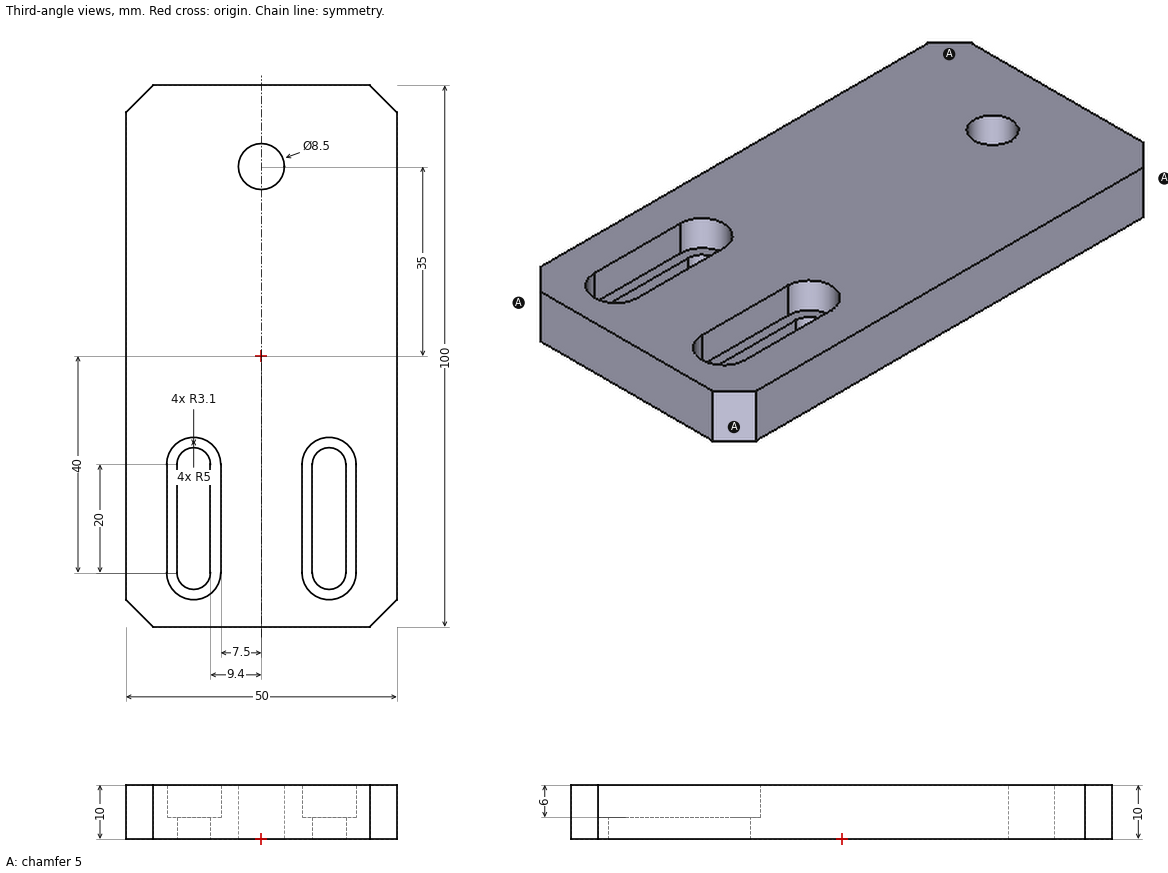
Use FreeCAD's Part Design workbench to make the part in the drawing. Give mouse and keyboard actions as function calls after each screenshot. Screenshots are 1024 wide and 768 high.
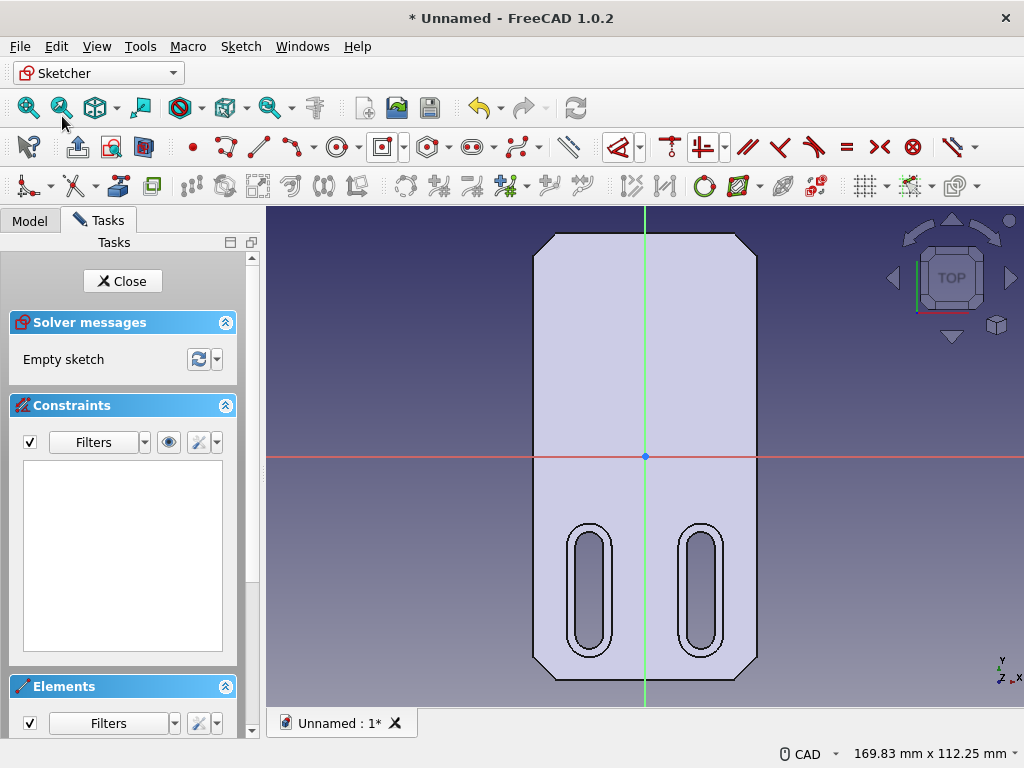
scroll(654, 281, up, 11)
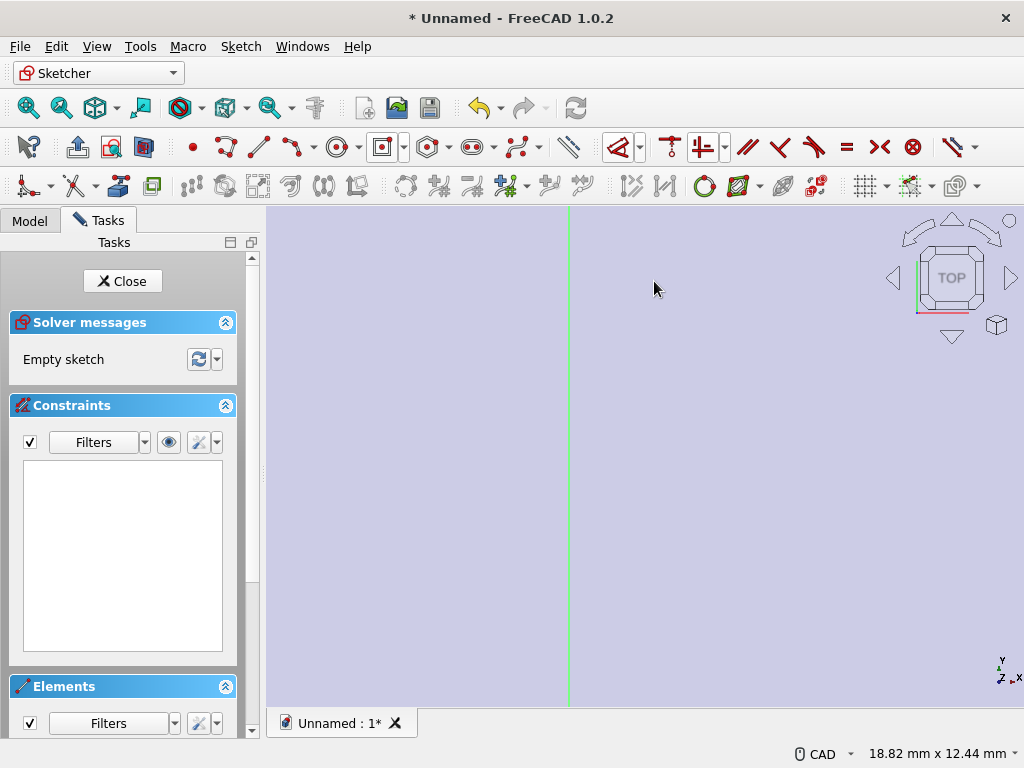
click(336, 148)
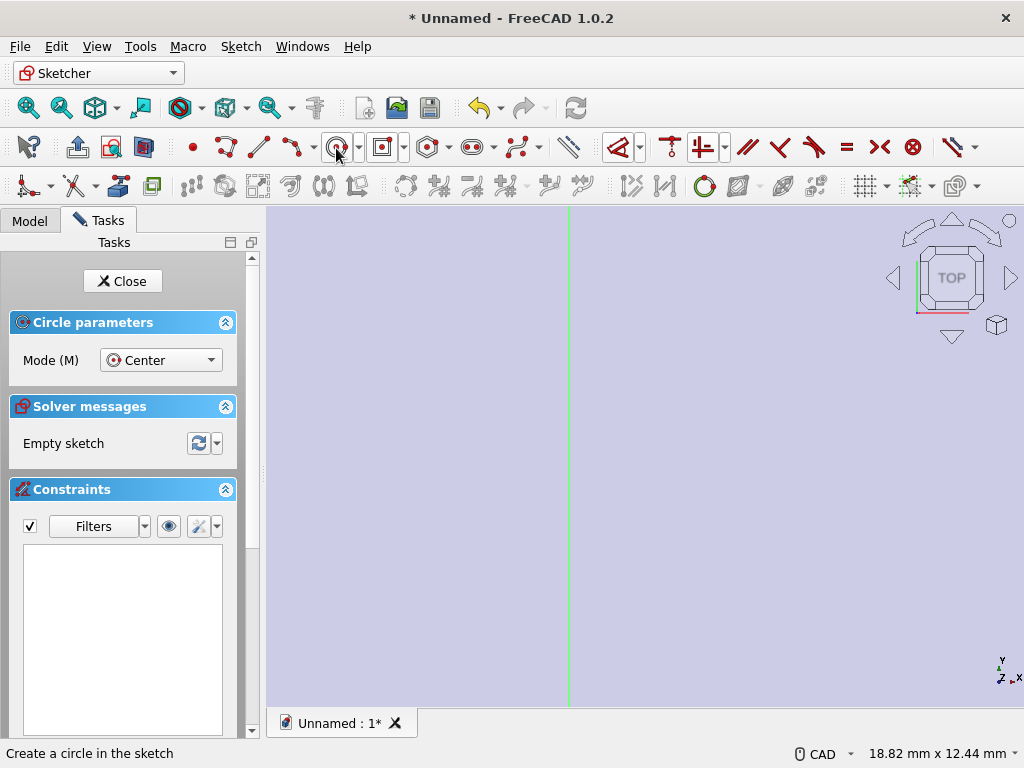
click(569, 454)
click(690, 333)
key(Escape)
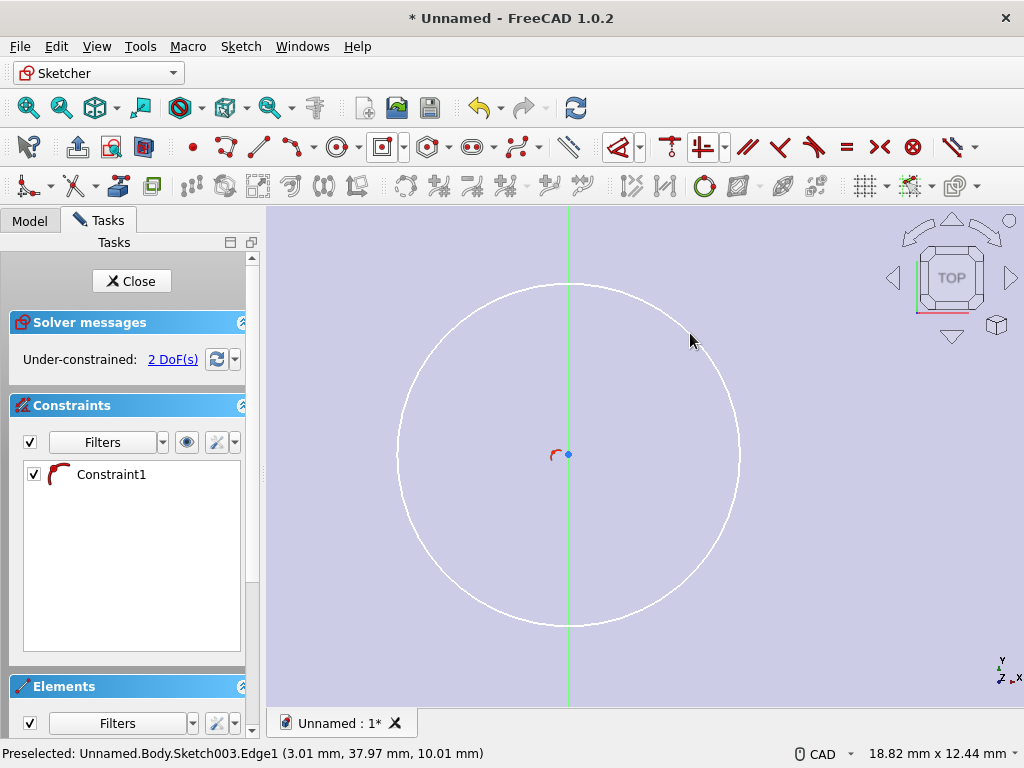
click(689, 333)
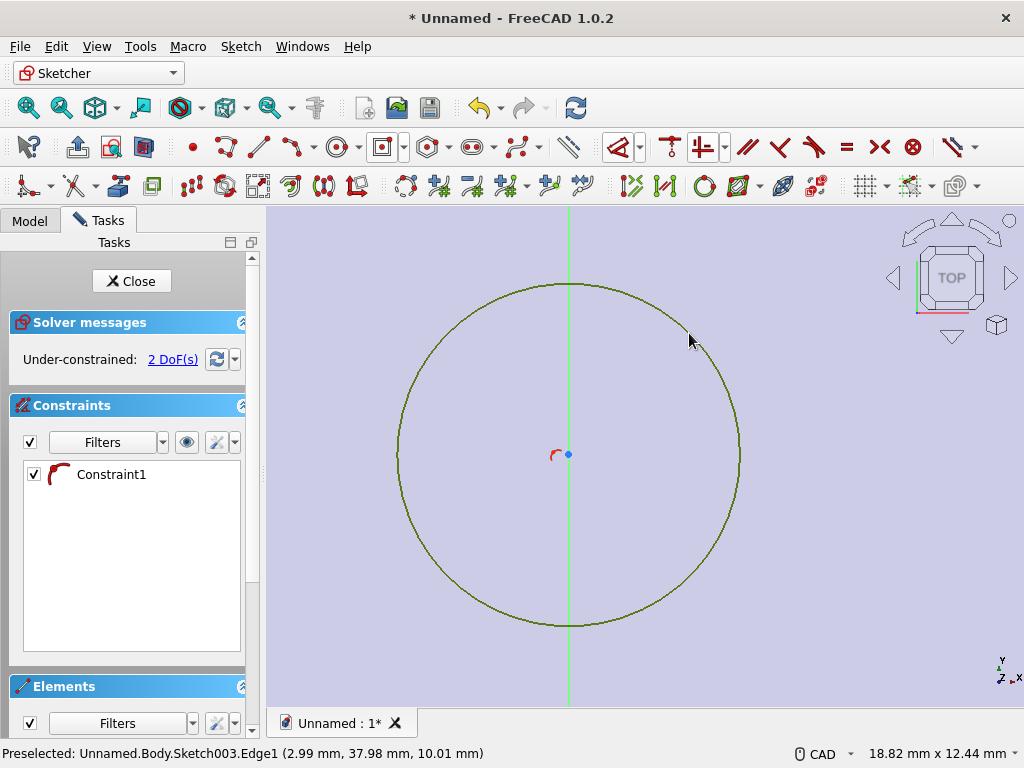
key(k)
key(o)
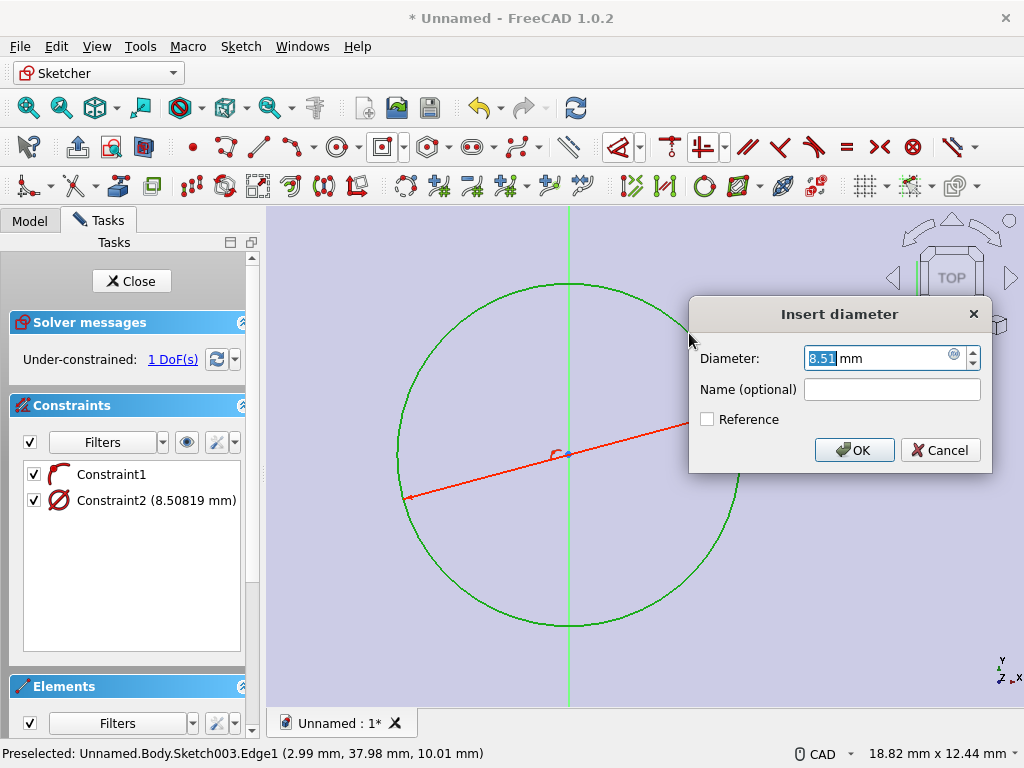
text(8.5)
key(Return)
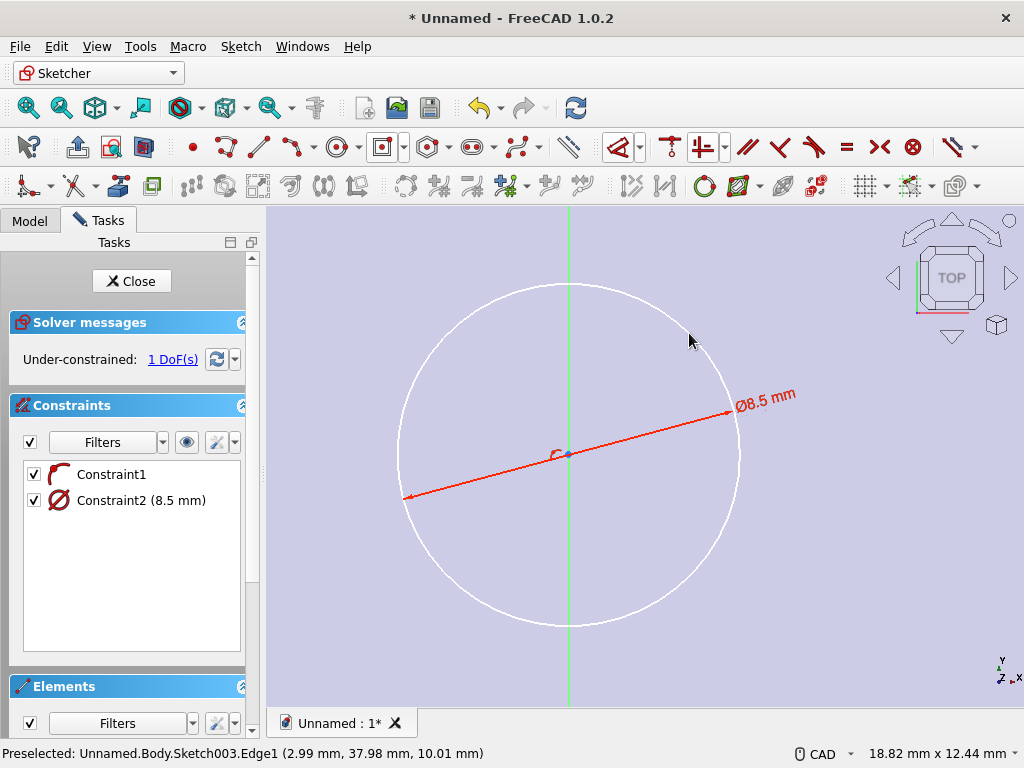
click(569, 455)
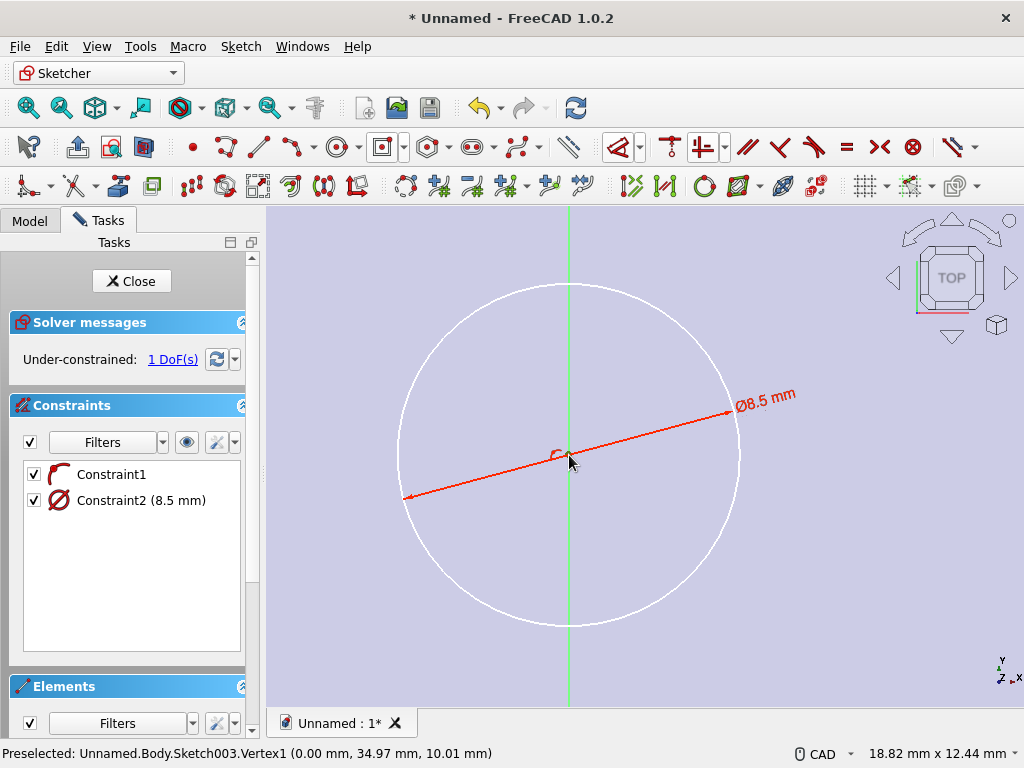
key(i)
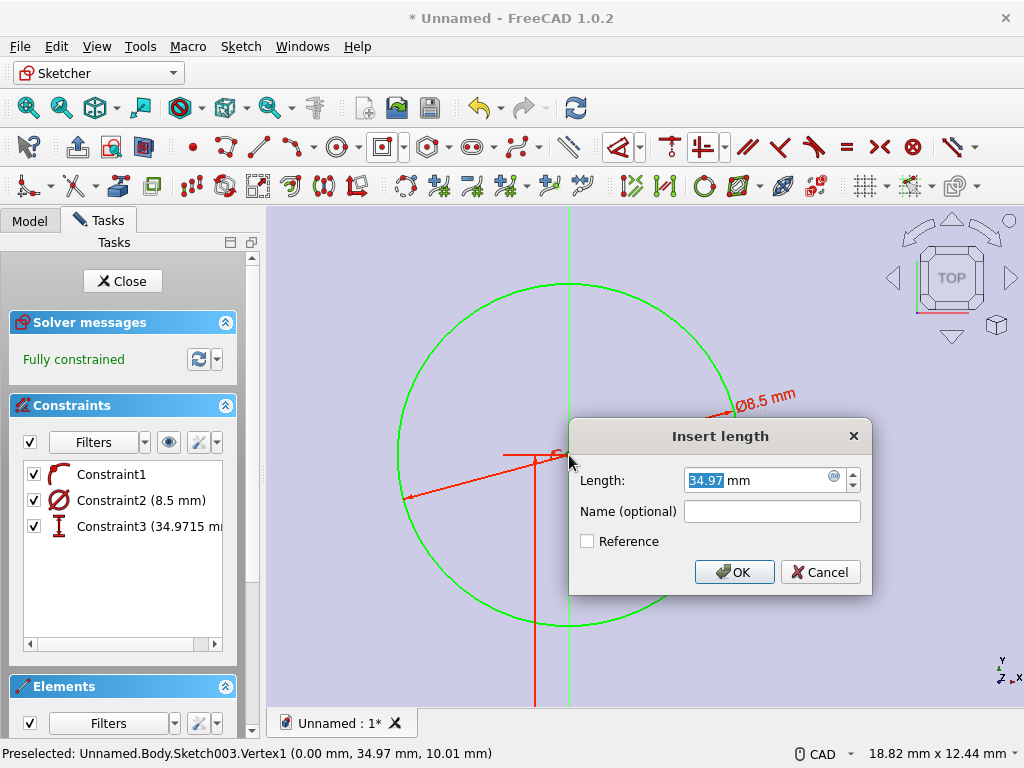
text(35)
key(Return)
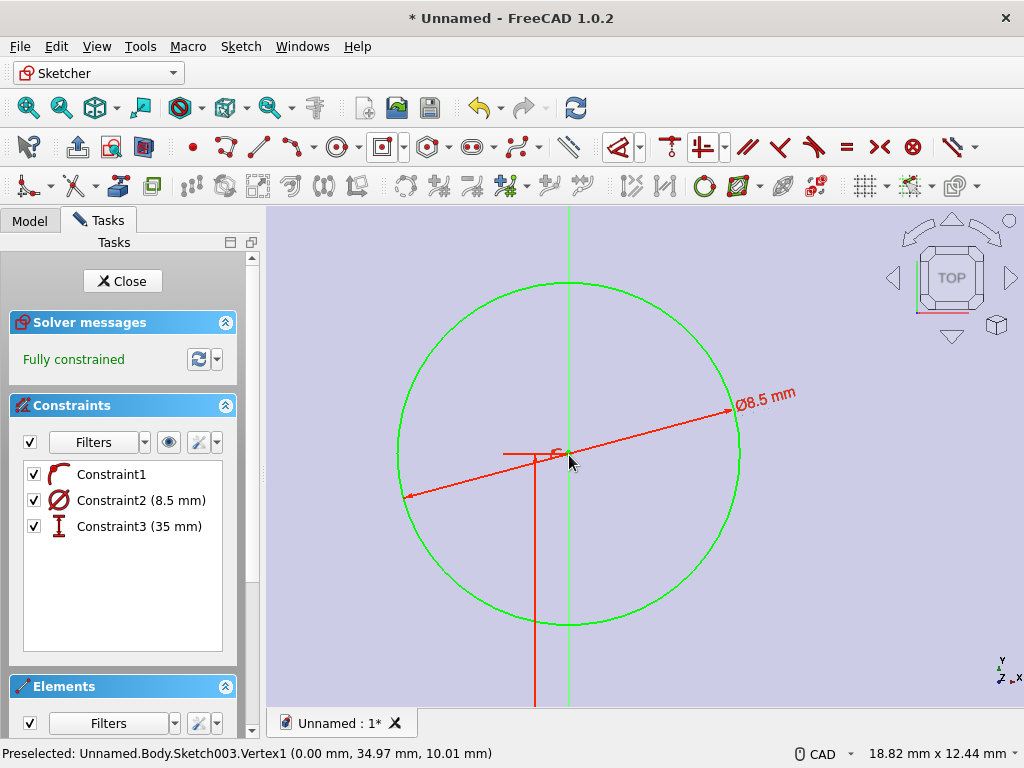
click(123, 281)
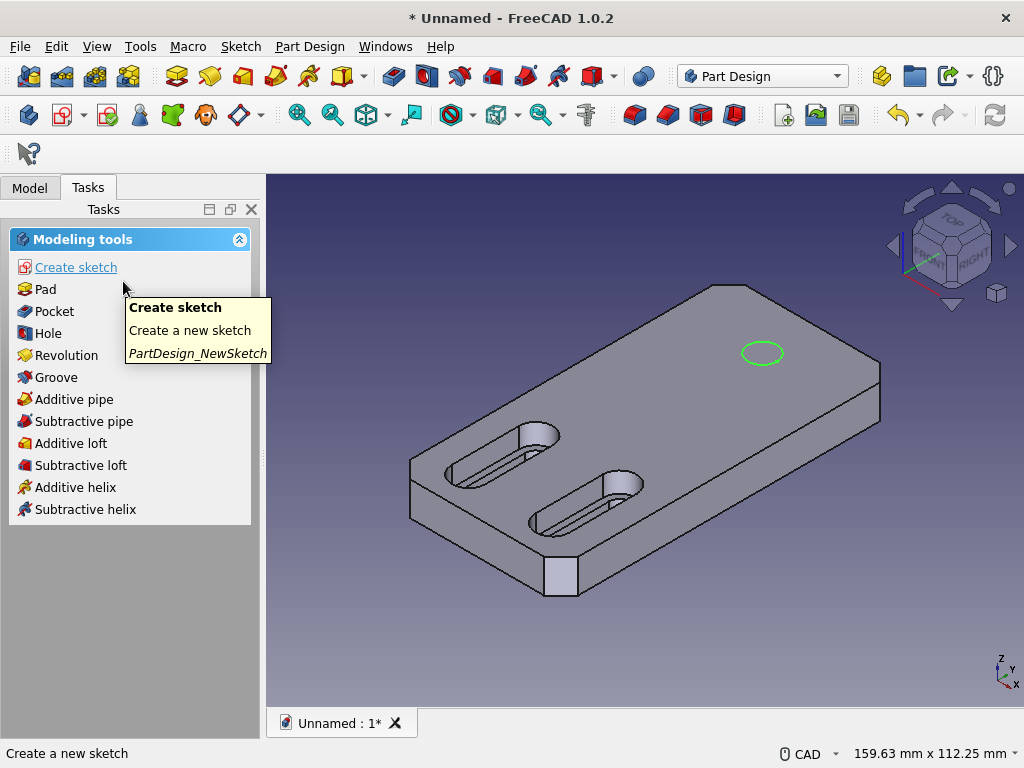
click(394, 76)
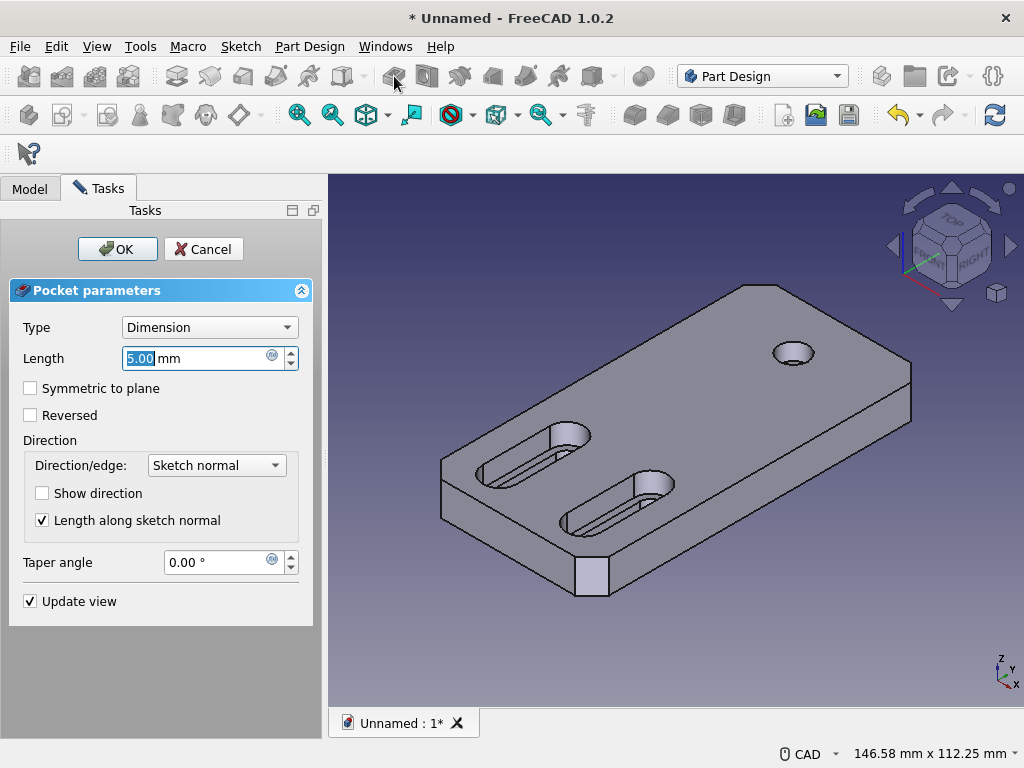
text(10)
key(Tab)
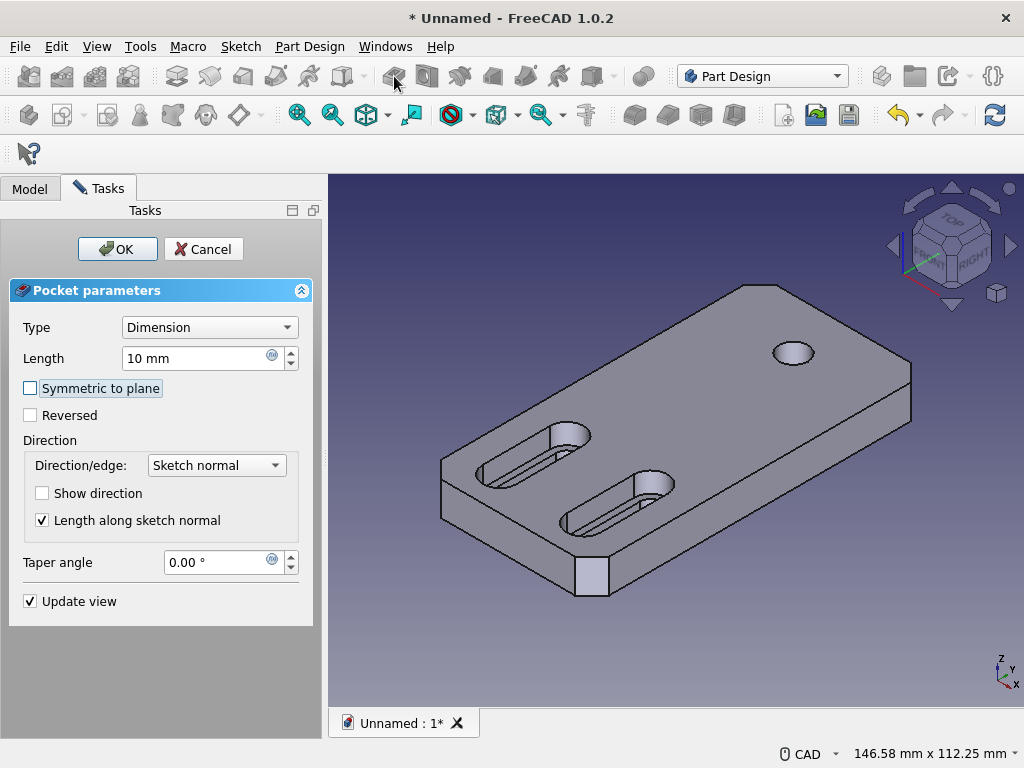
click(118, 249)